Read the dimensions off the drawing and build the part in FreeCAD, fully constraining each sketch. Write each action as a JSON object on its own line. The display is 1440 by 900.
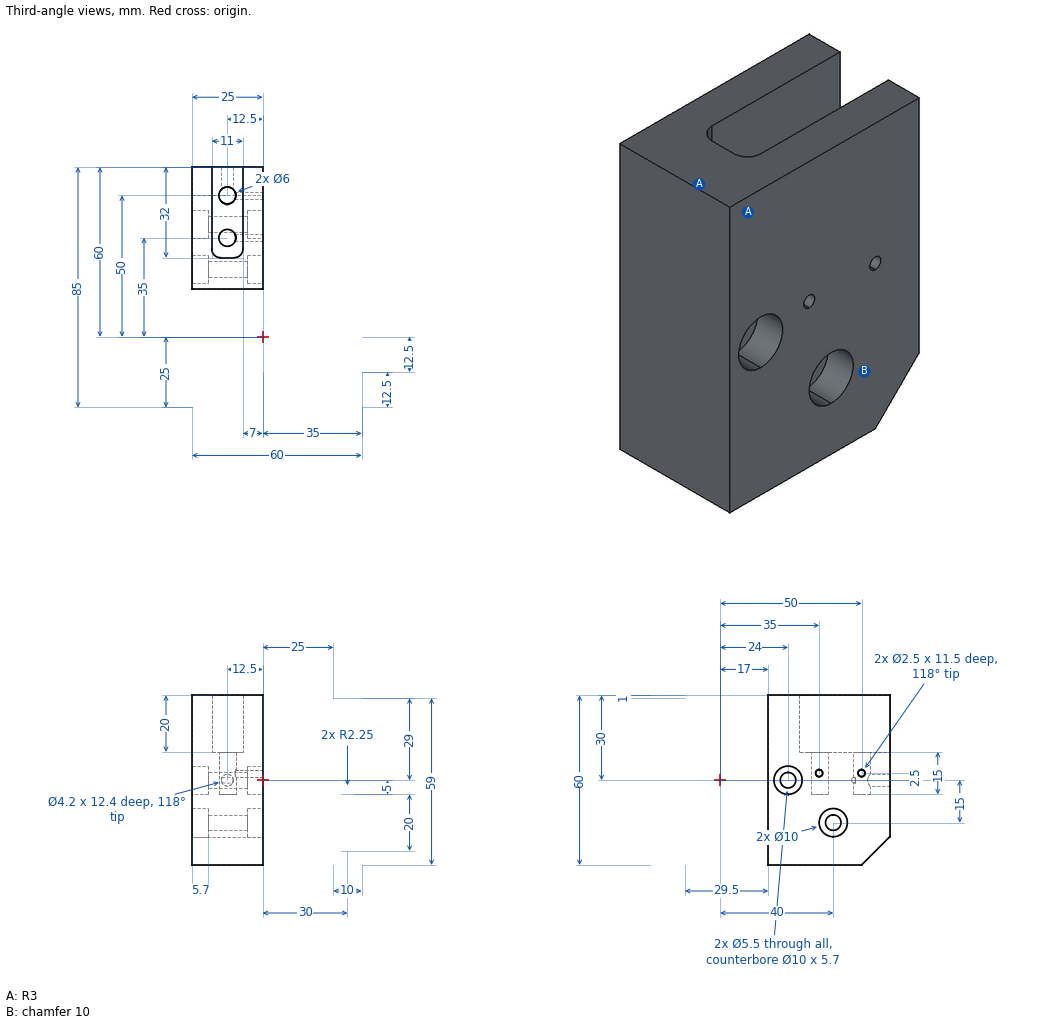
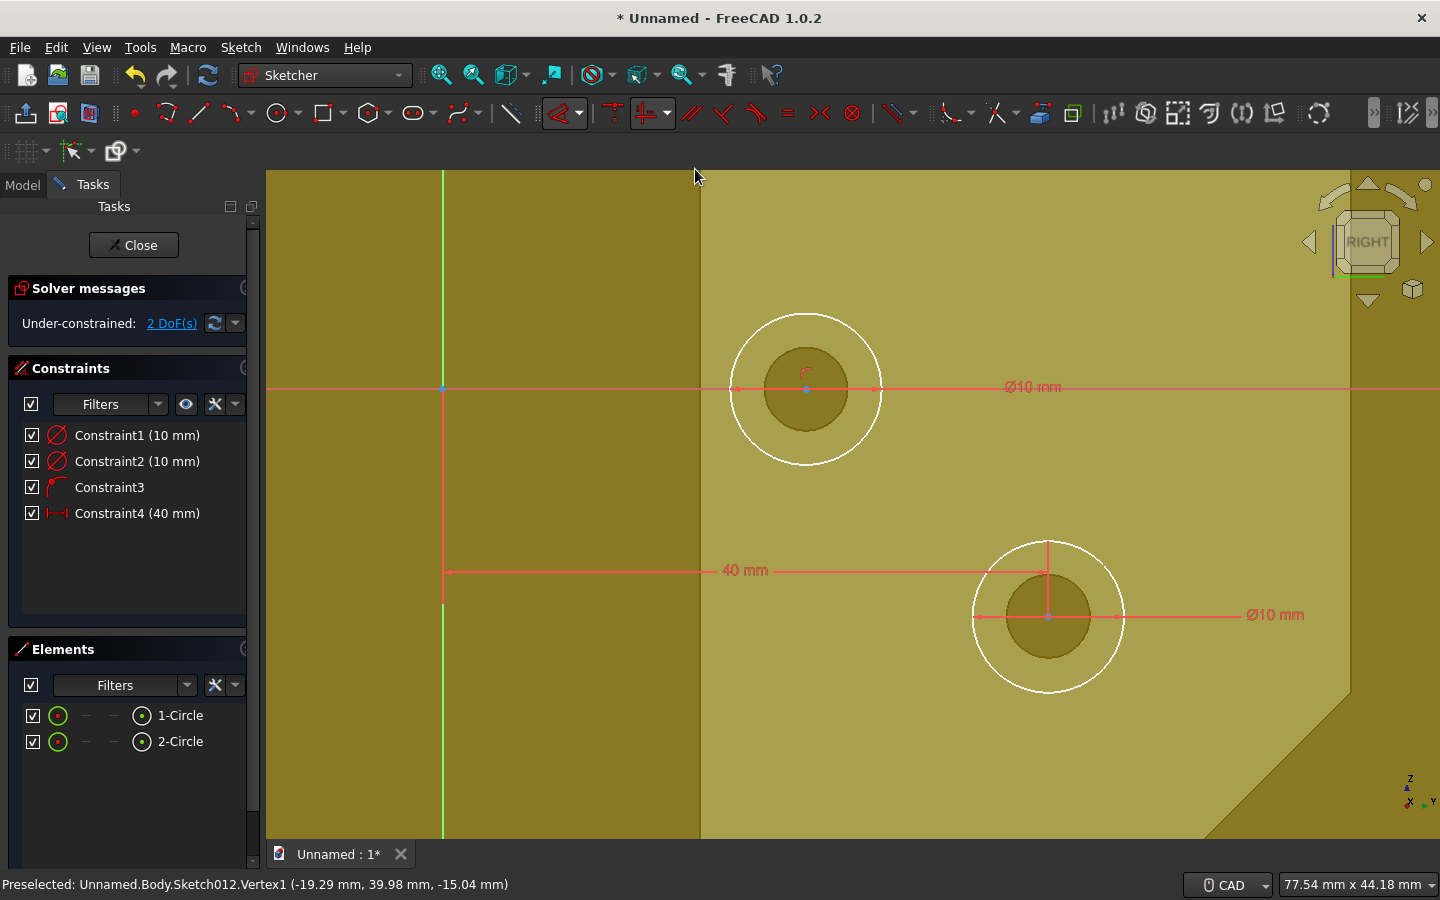
{"action": "left_click", "coordinate": [1048, 617]}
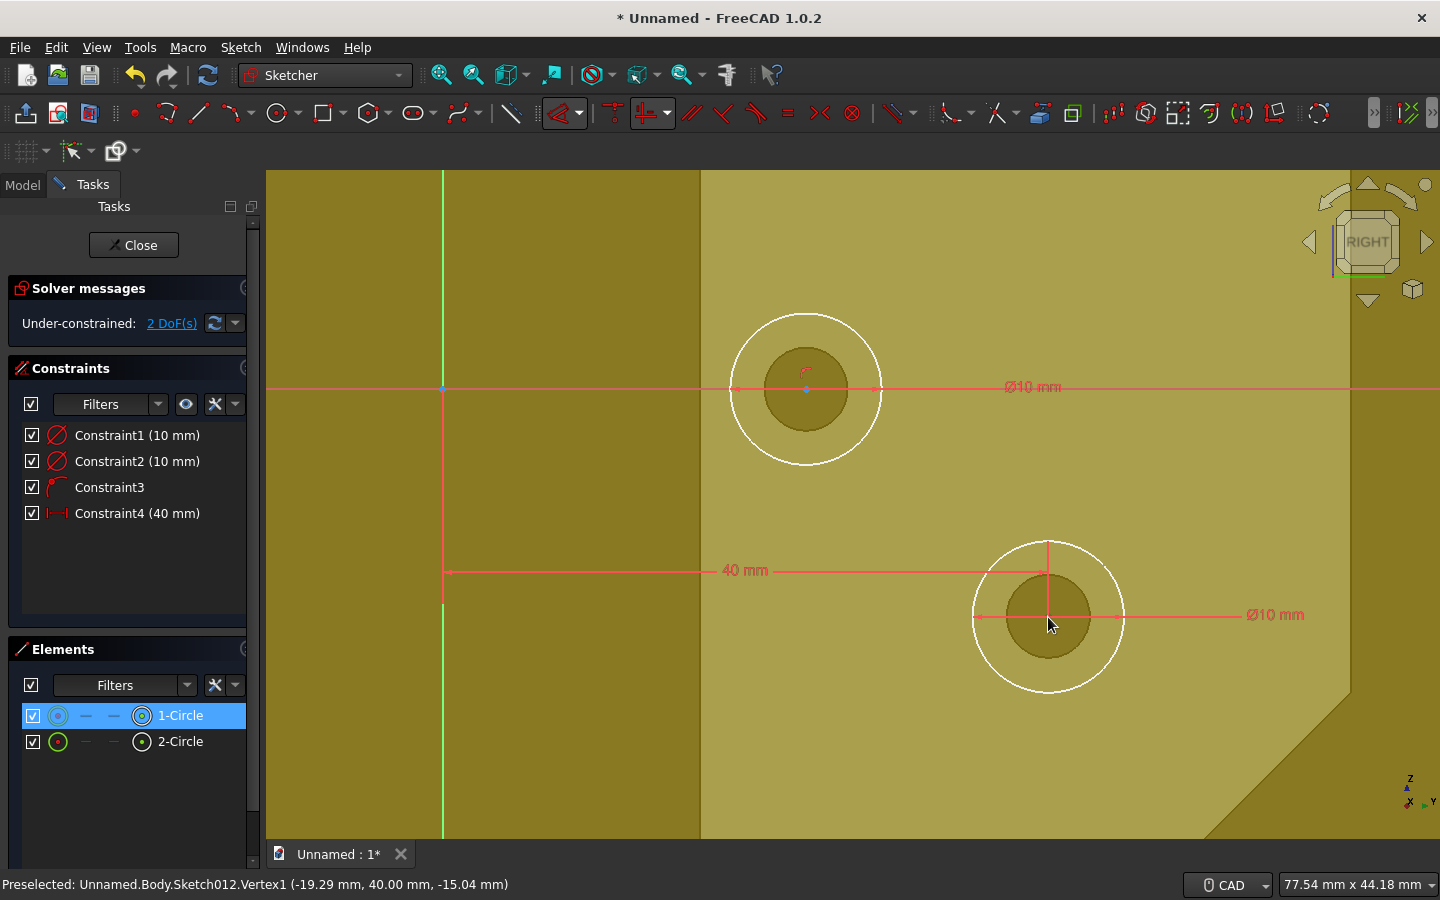
{"action": "left_click", "coordinate": [582, 114]}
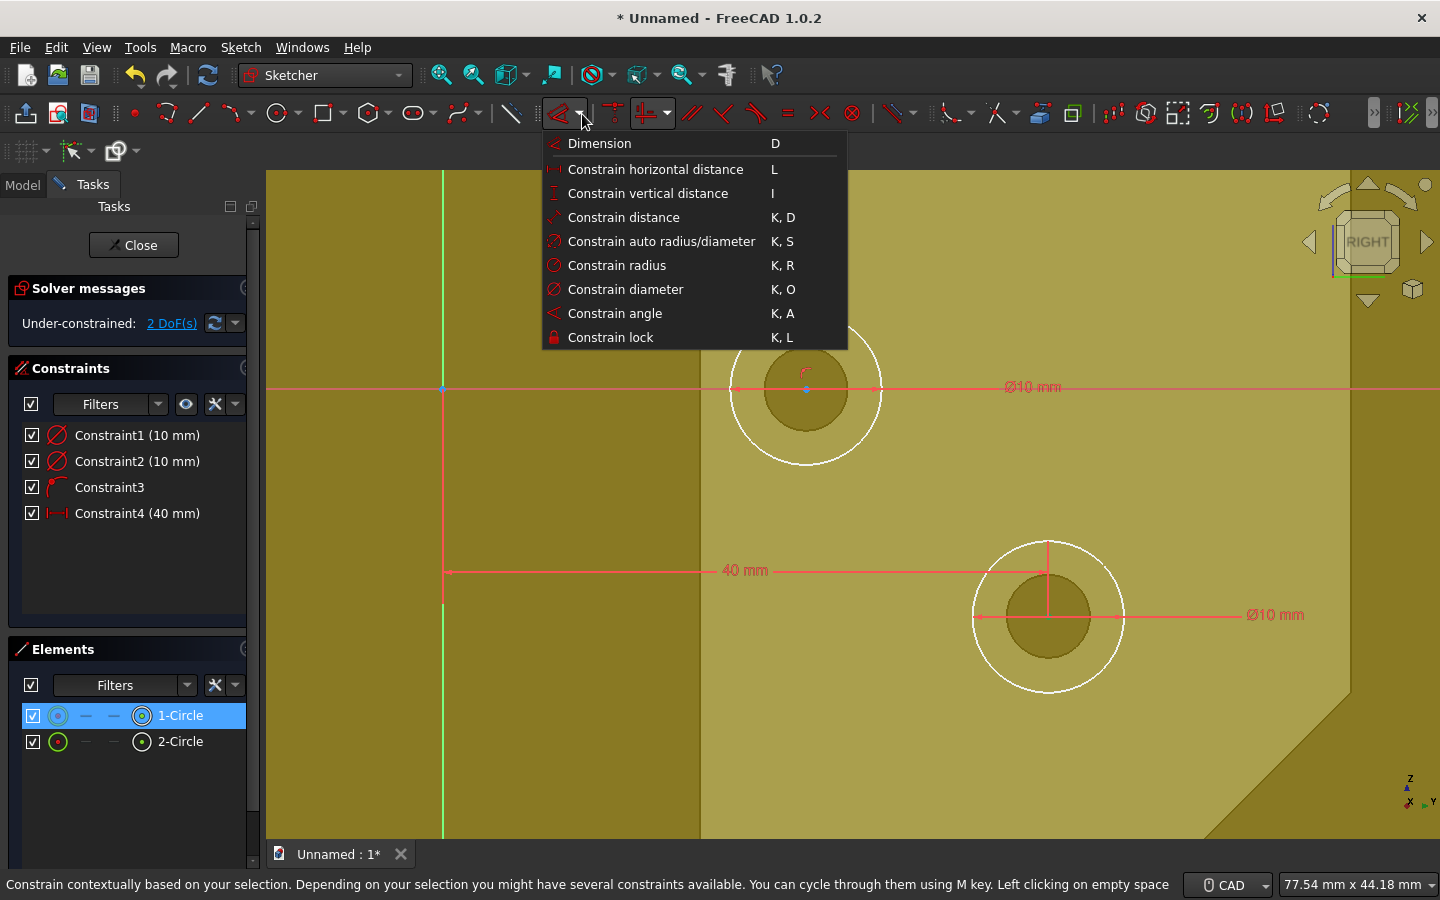
{"action": "left_click", "coordinate": [695, 193]}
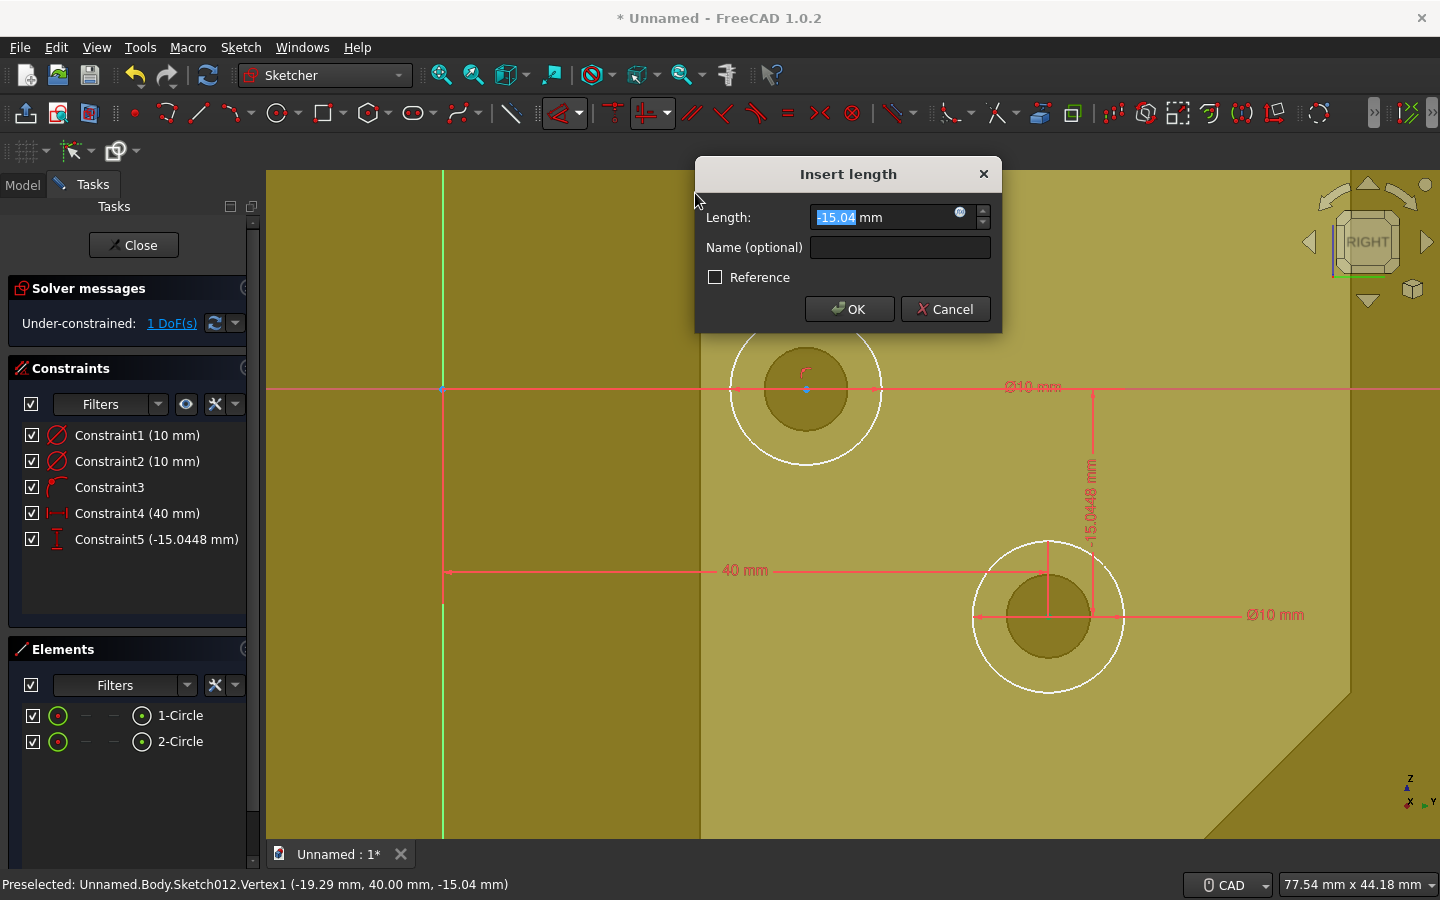
{"action": "type", "text": "-15"}
{"action": "key", "text": "Return"}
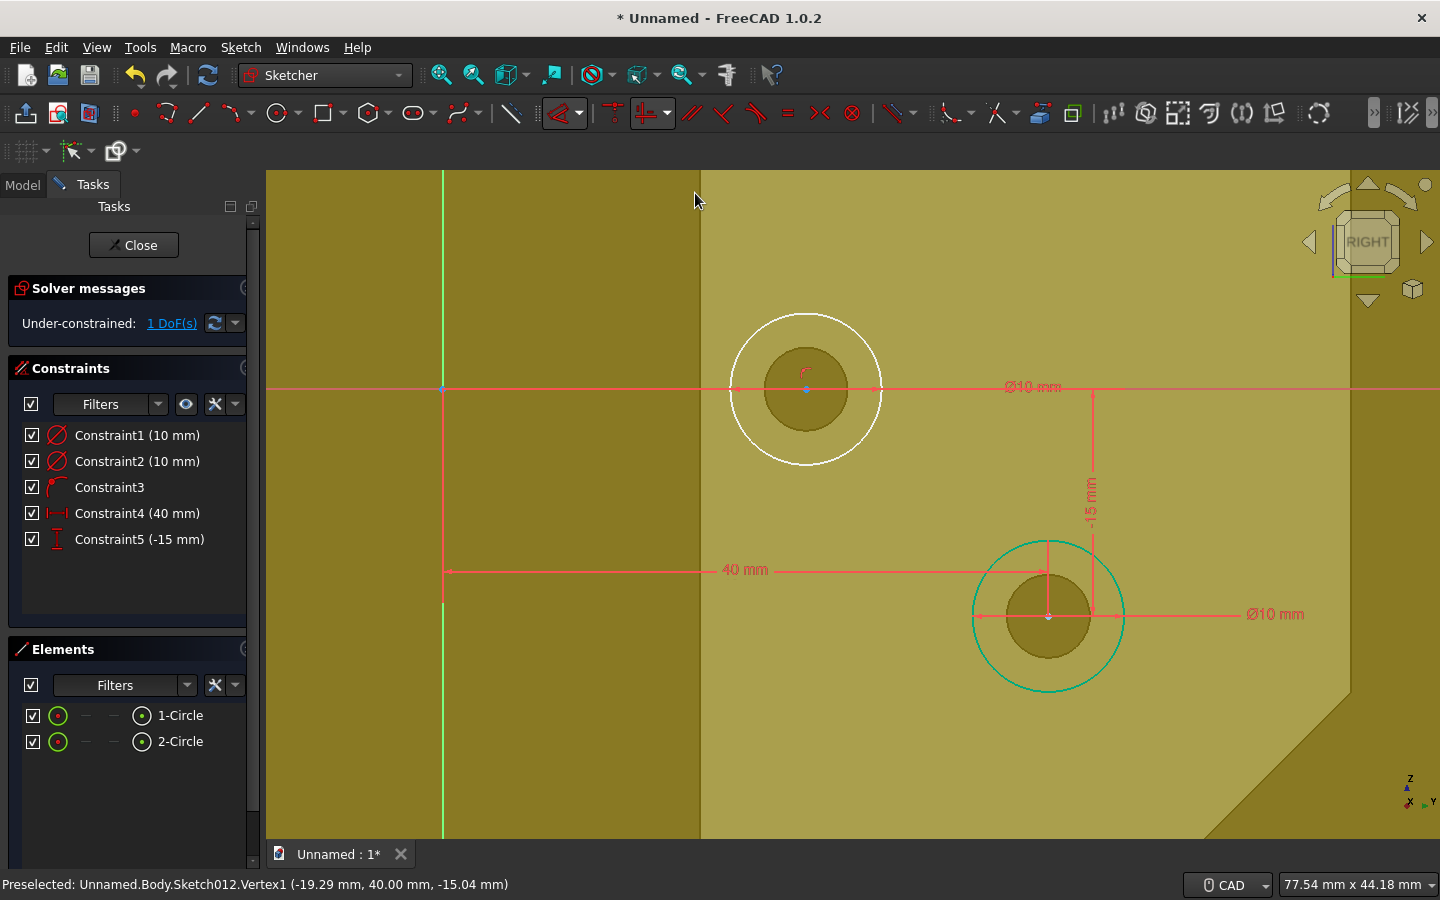
{"action": "left_click", "coordinate": [806, 389]}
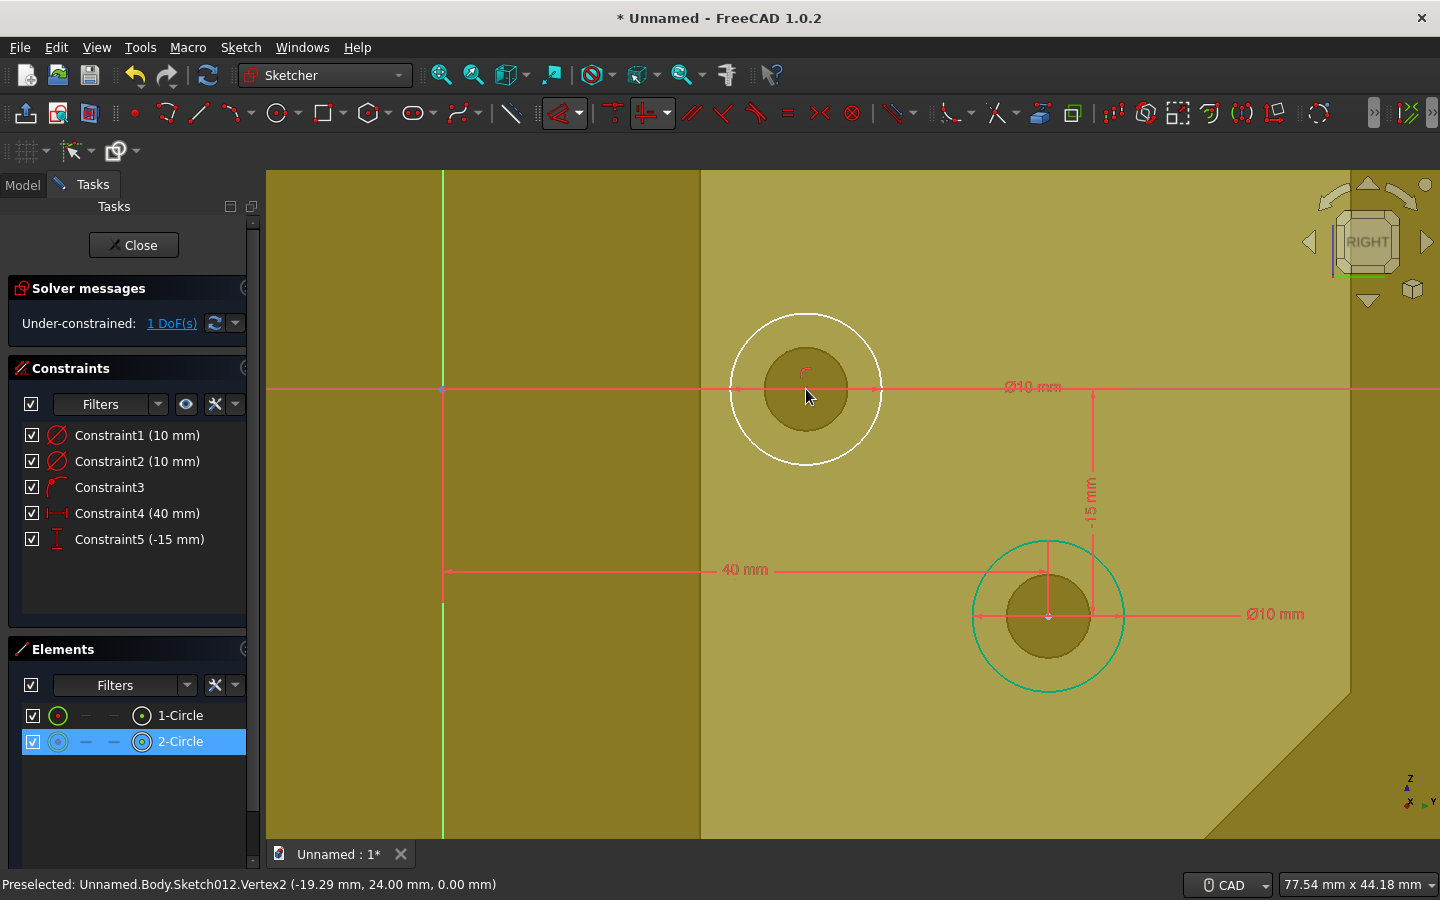
{"action": "left_click", "coordinate": [582, 114]}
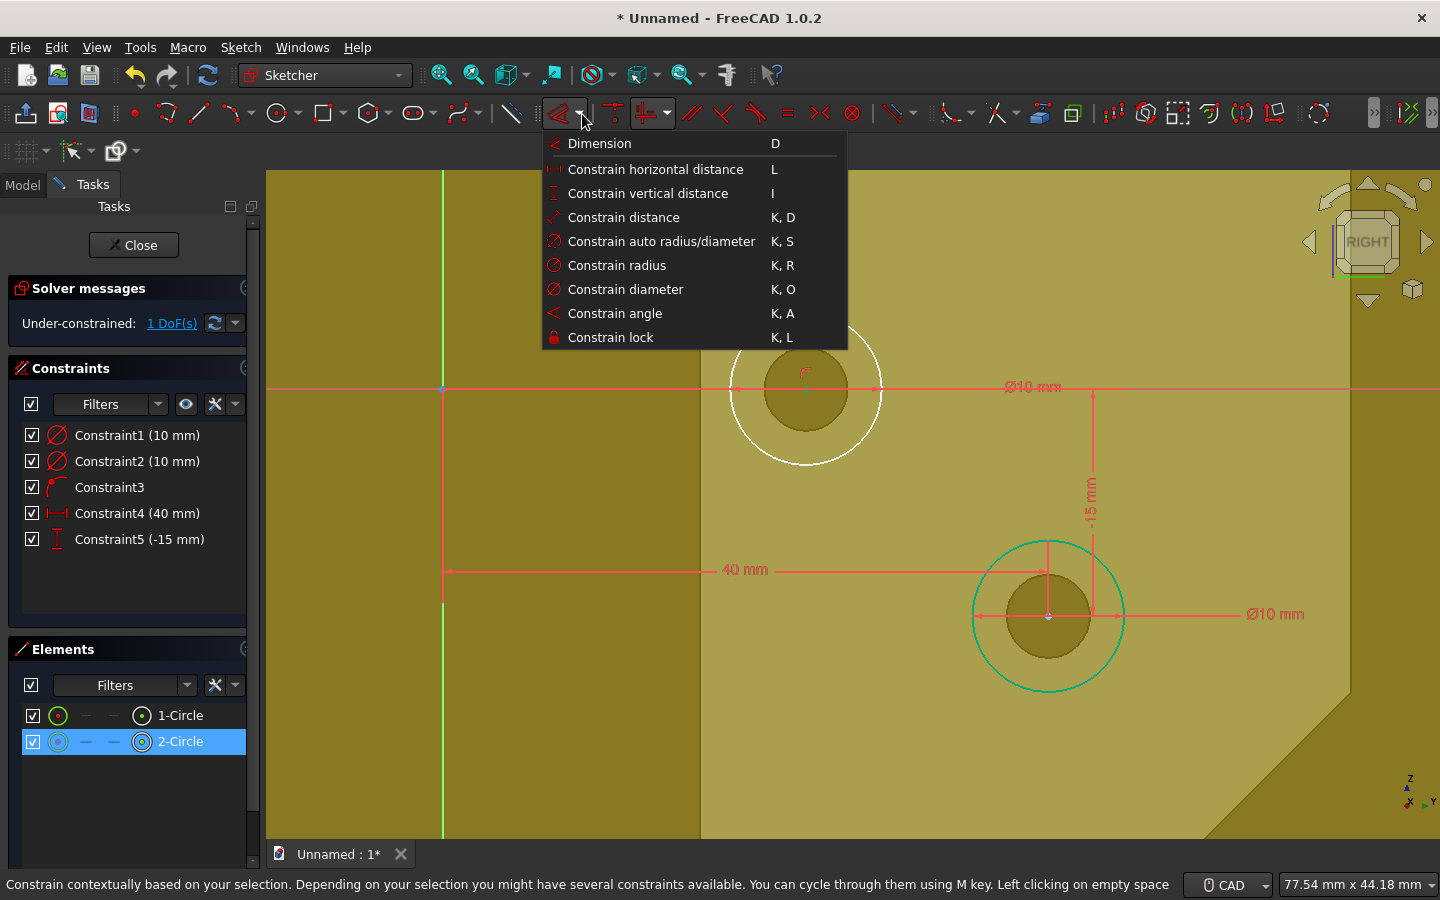
{"action": "left_click", "coordinate": [695, 169]}